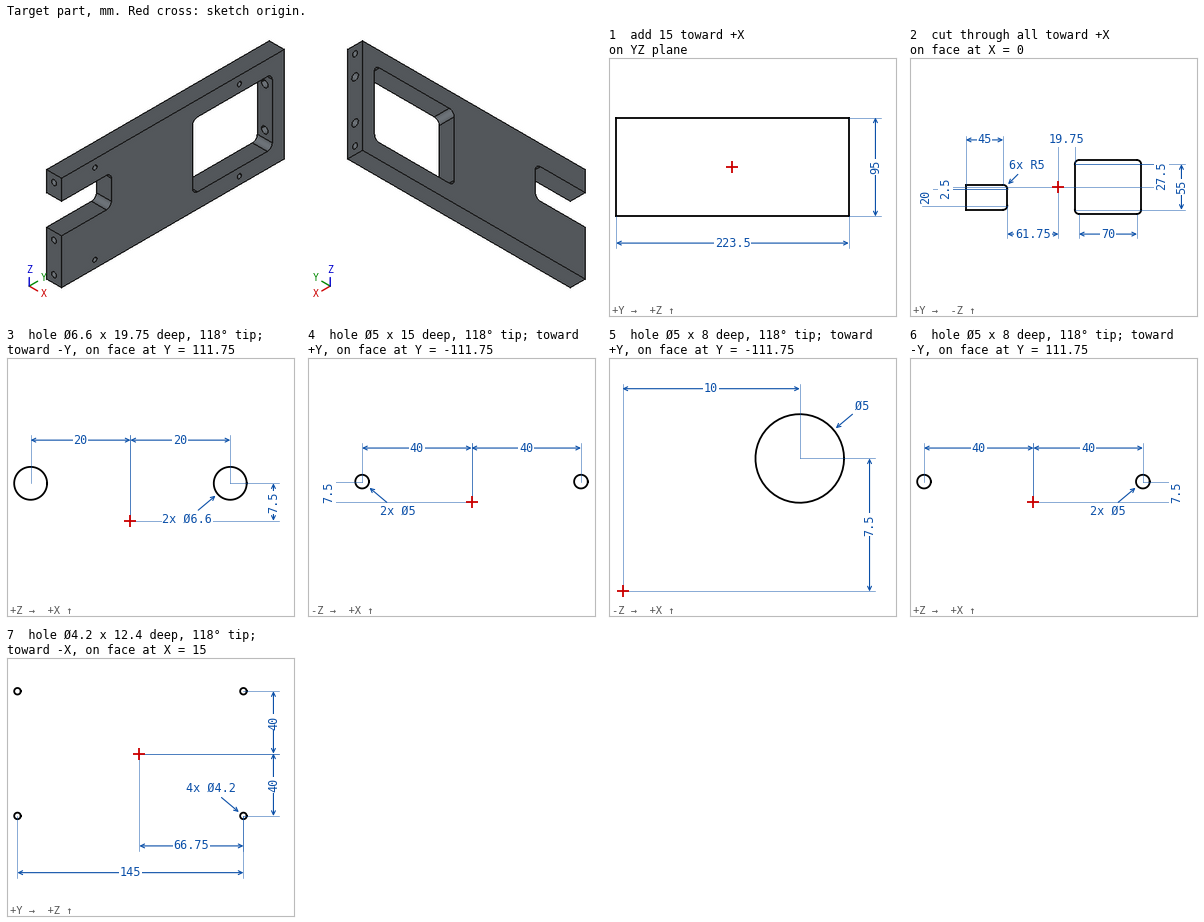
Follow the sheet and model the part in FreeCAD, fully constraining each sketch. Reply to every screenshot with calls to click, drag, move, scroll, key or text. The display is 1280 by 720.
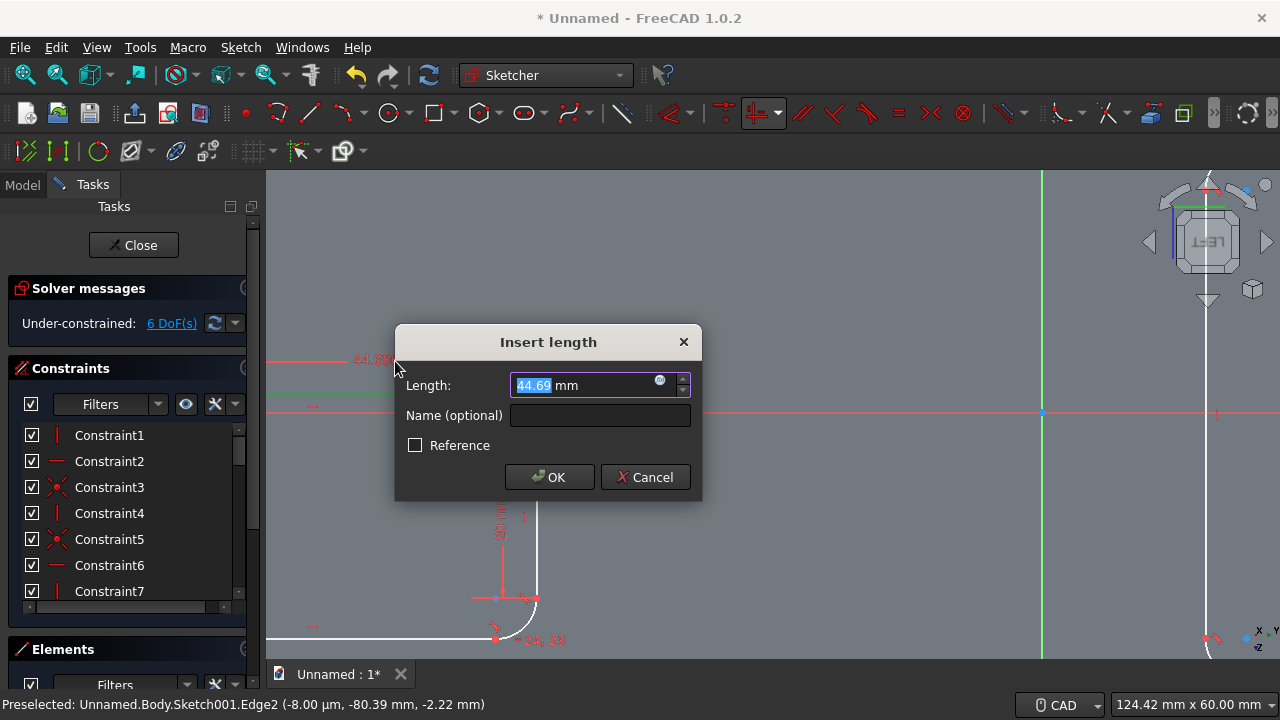
text(45)
key(Return)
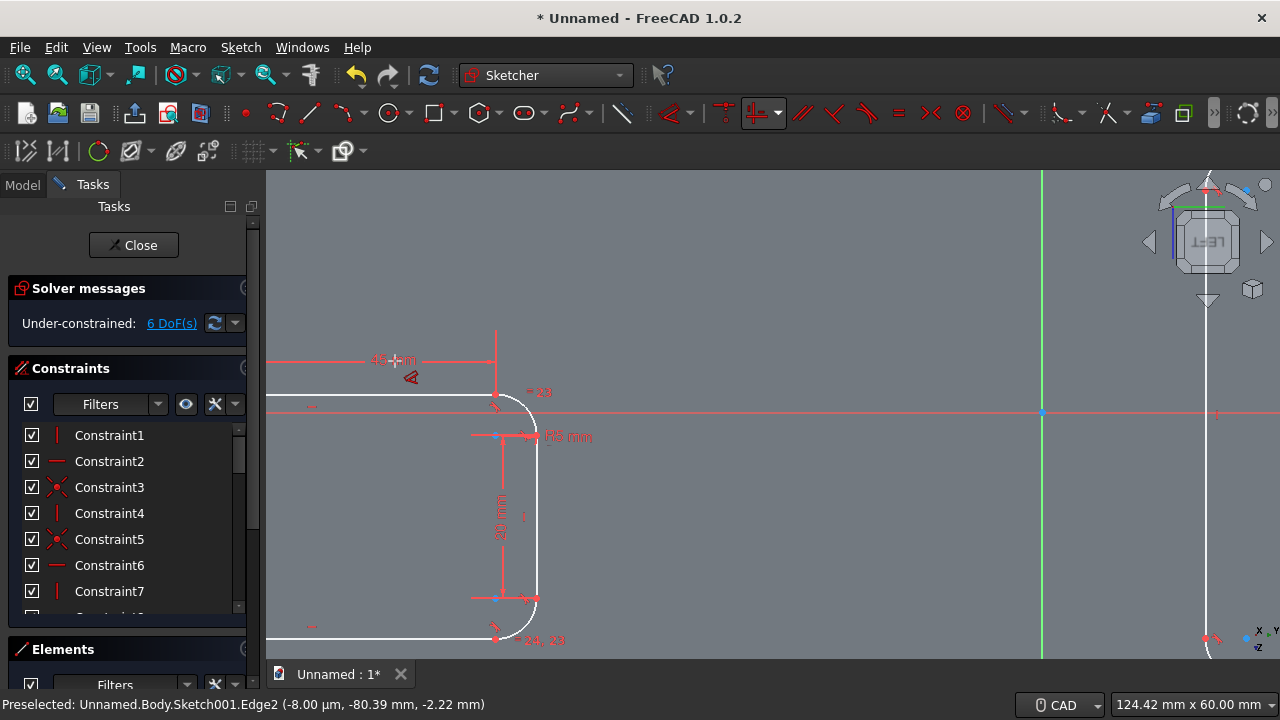
scroll(536, 416, down, 5)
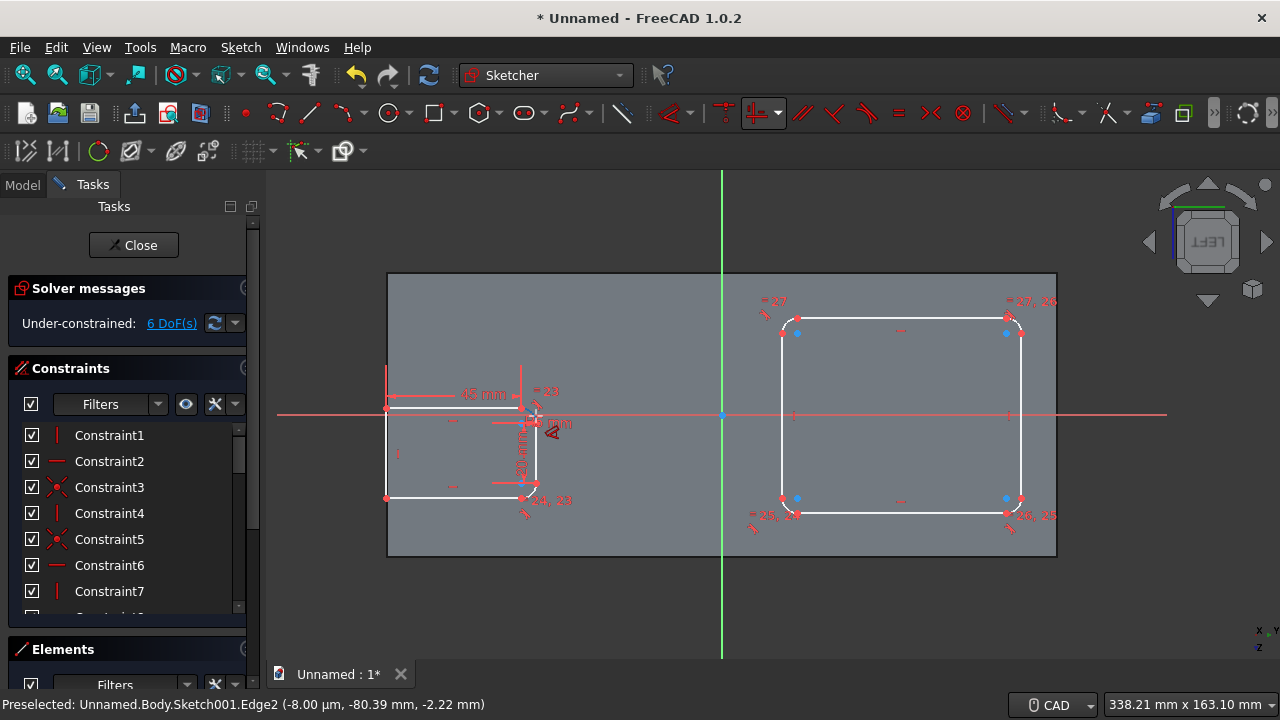
click(782, 383)
click(816, 378)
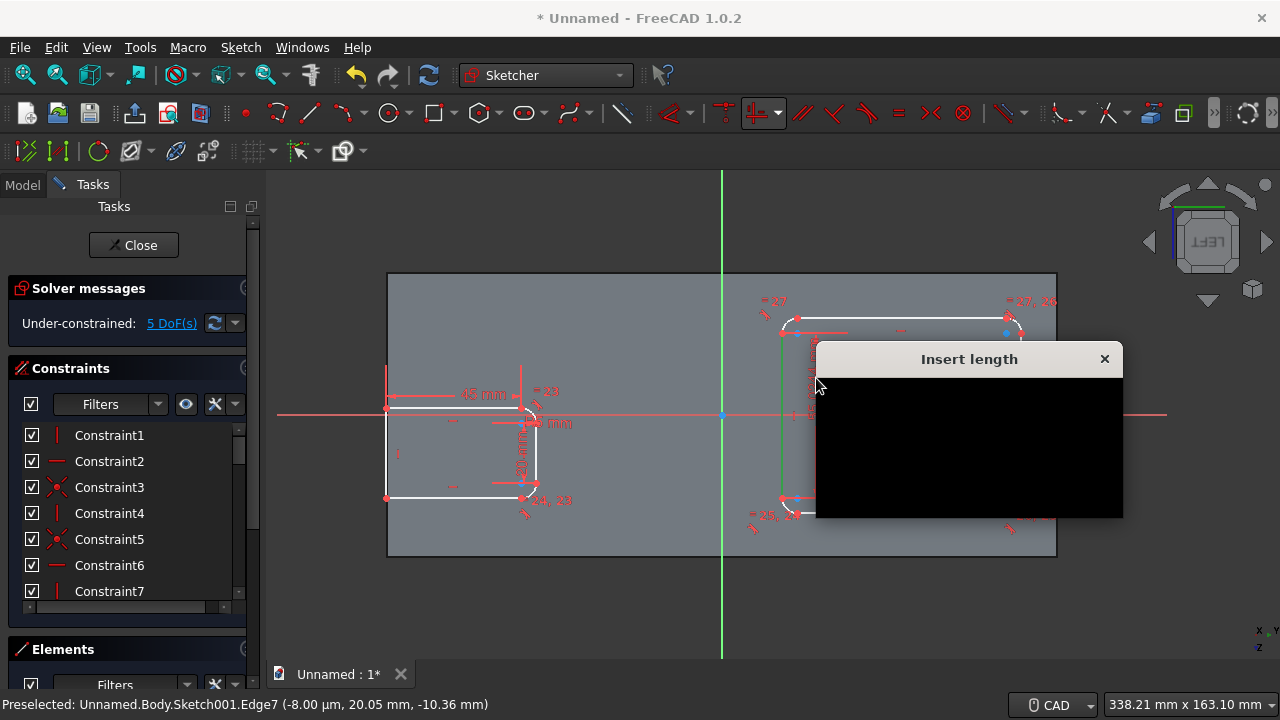
text(55)
key(Return)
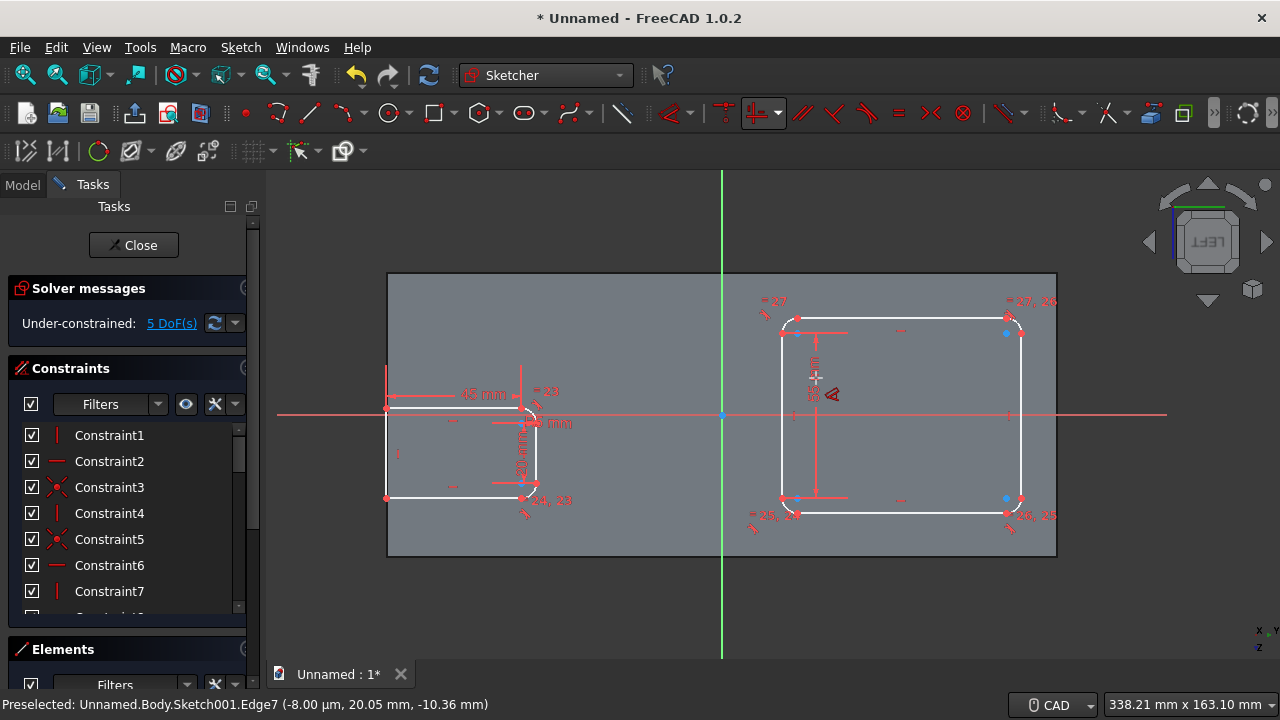
click(860, 513)
click(902, 547)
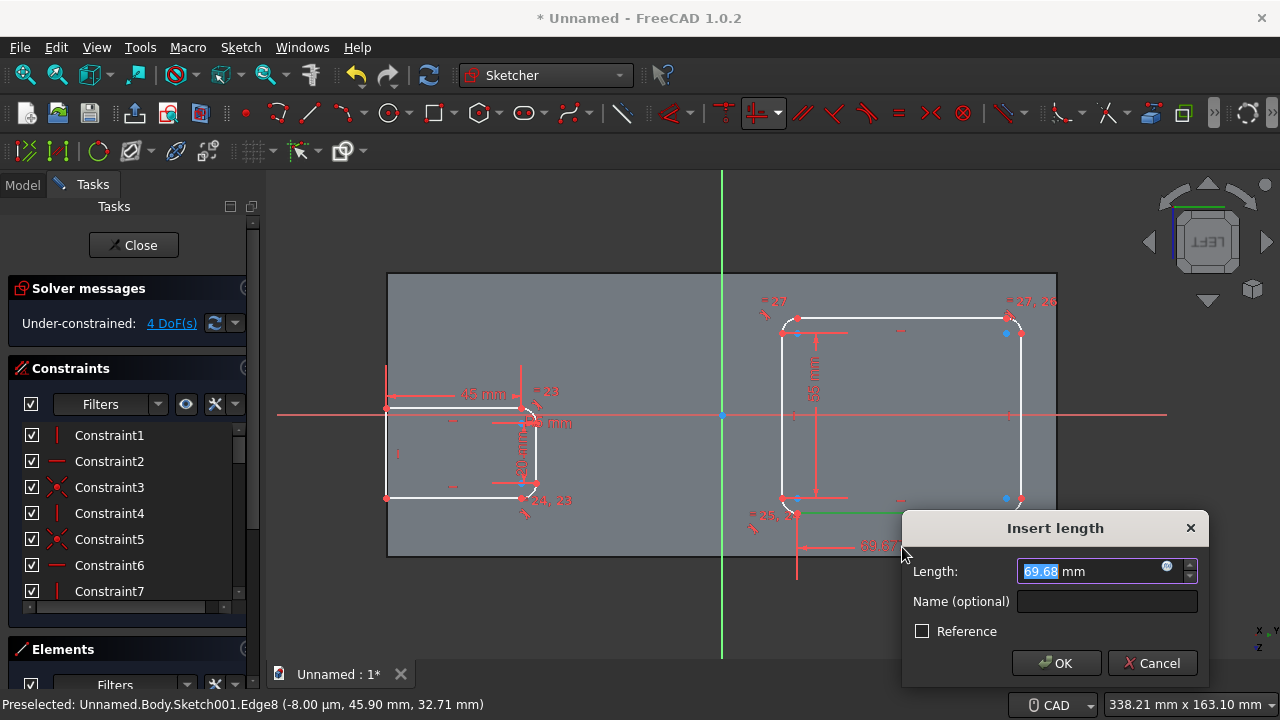
text(70)
key(Return)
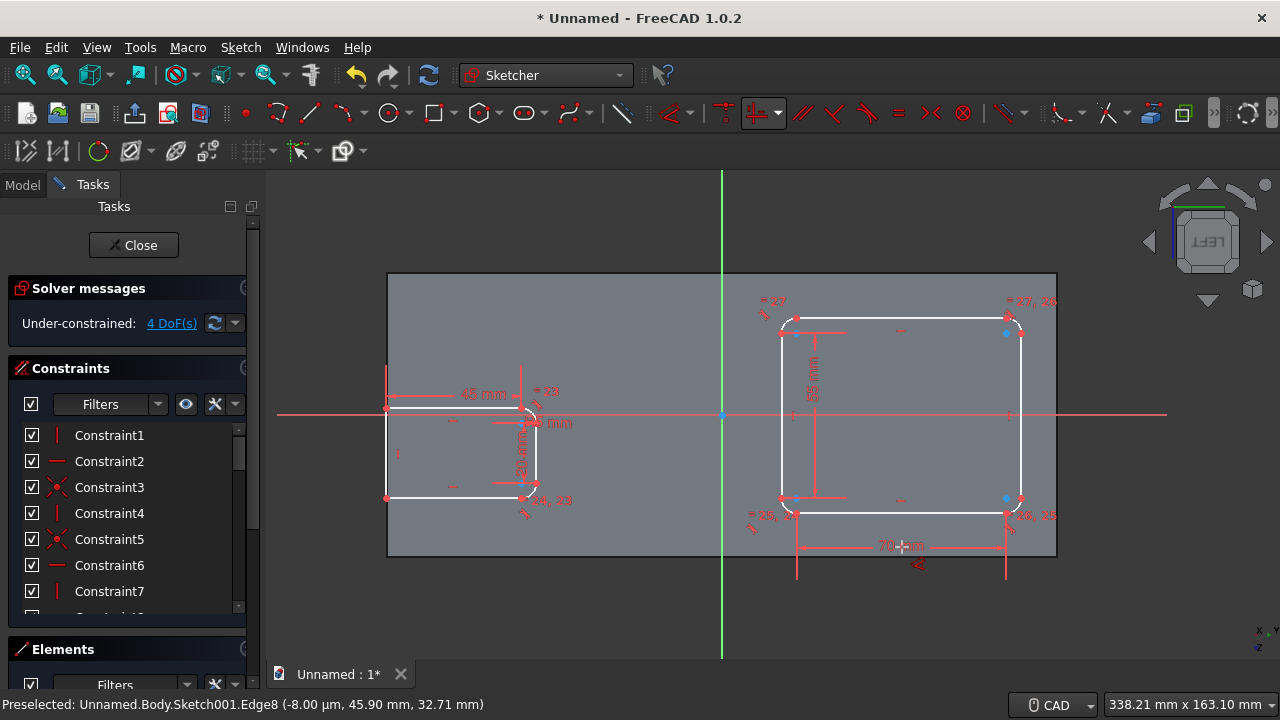
scroll(536, 423, up, 9)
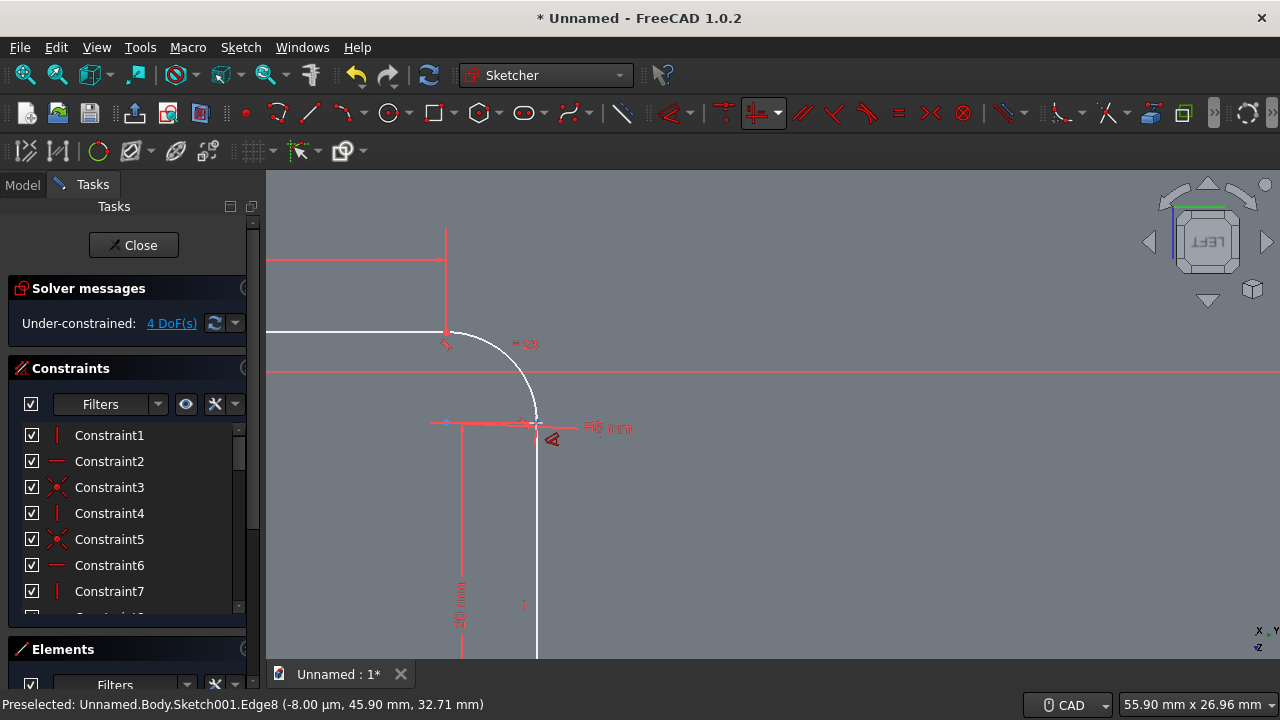
click(537, 423)
click(503, 398)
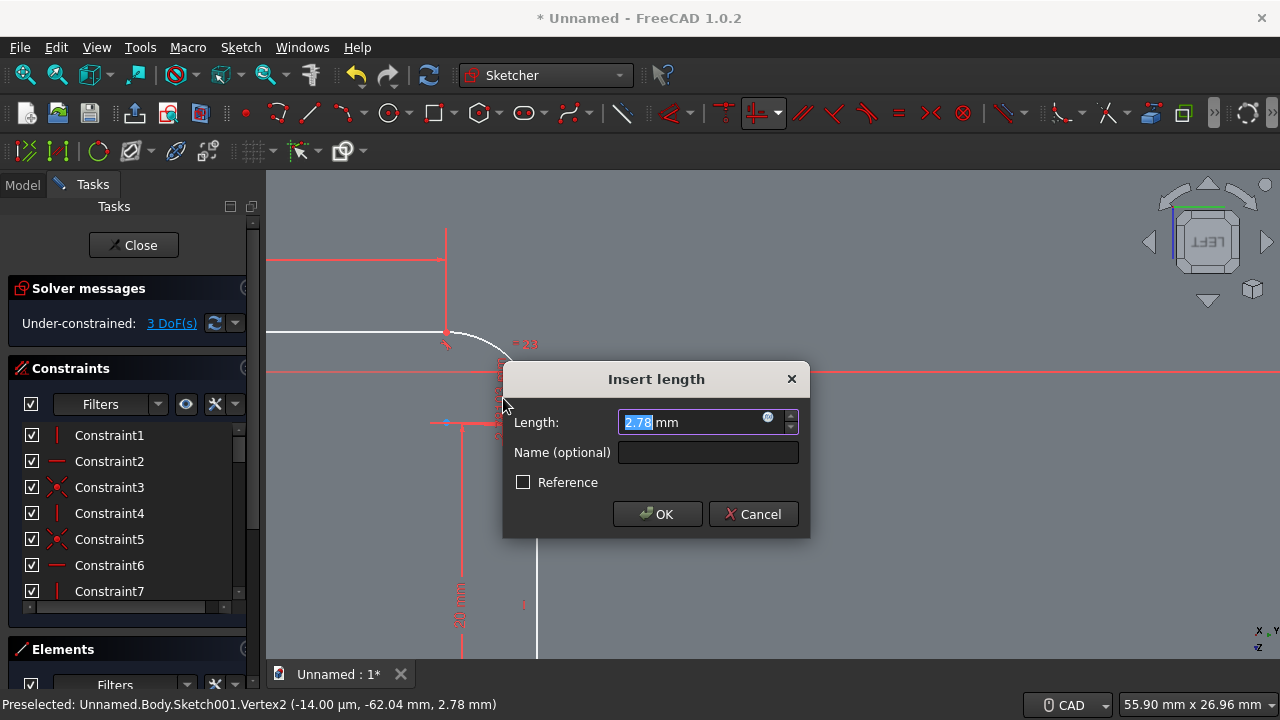
text(2.5)
key(Return)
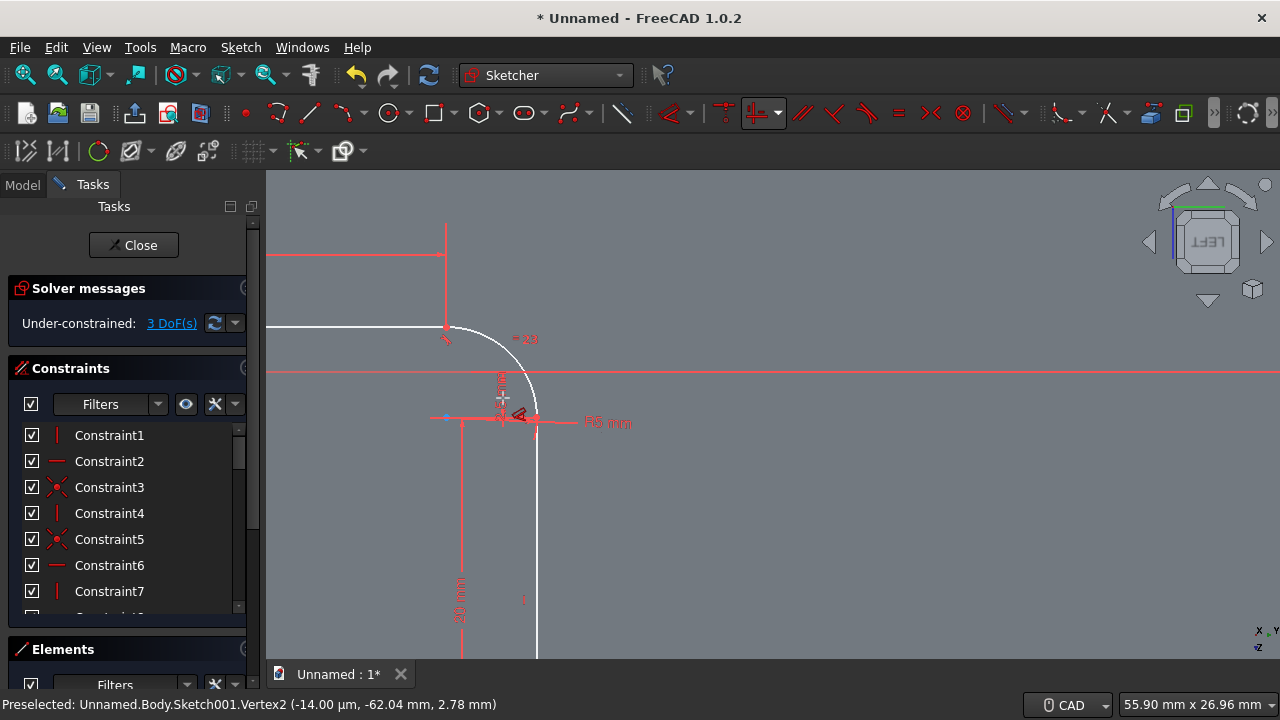
scroll(536, 423, down, 9)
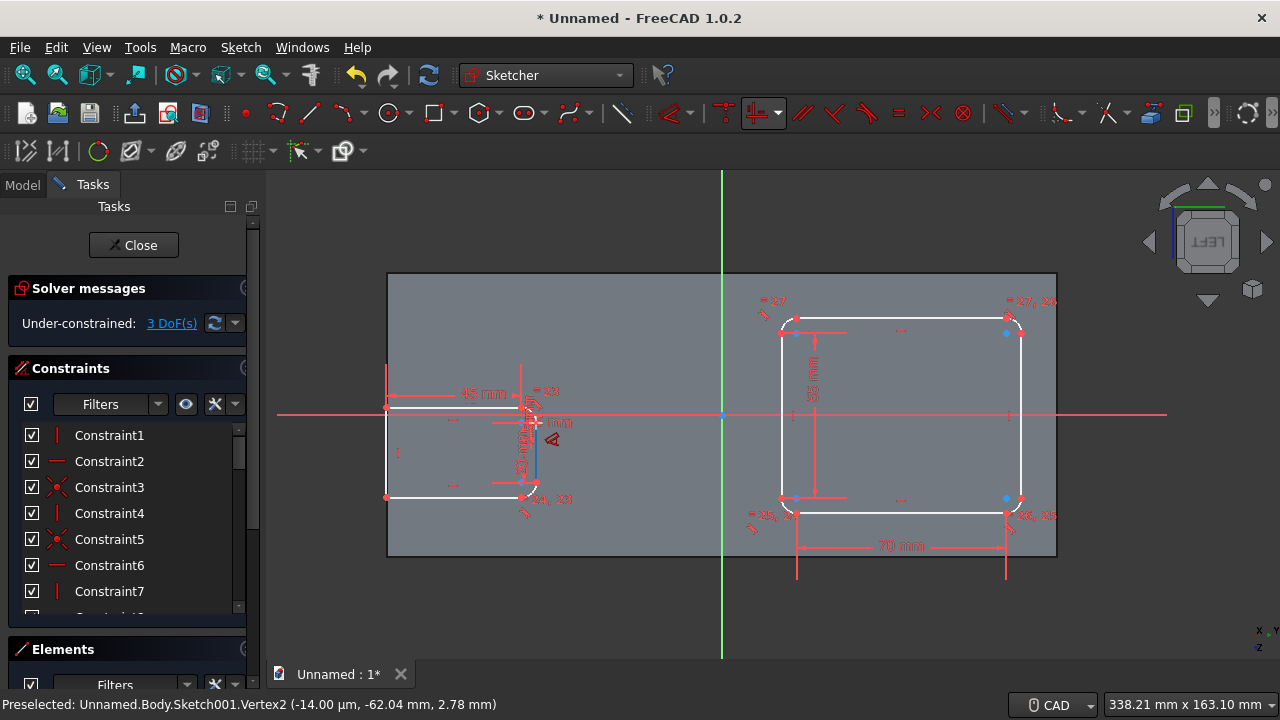
click(782, 333)
click(816, 355)